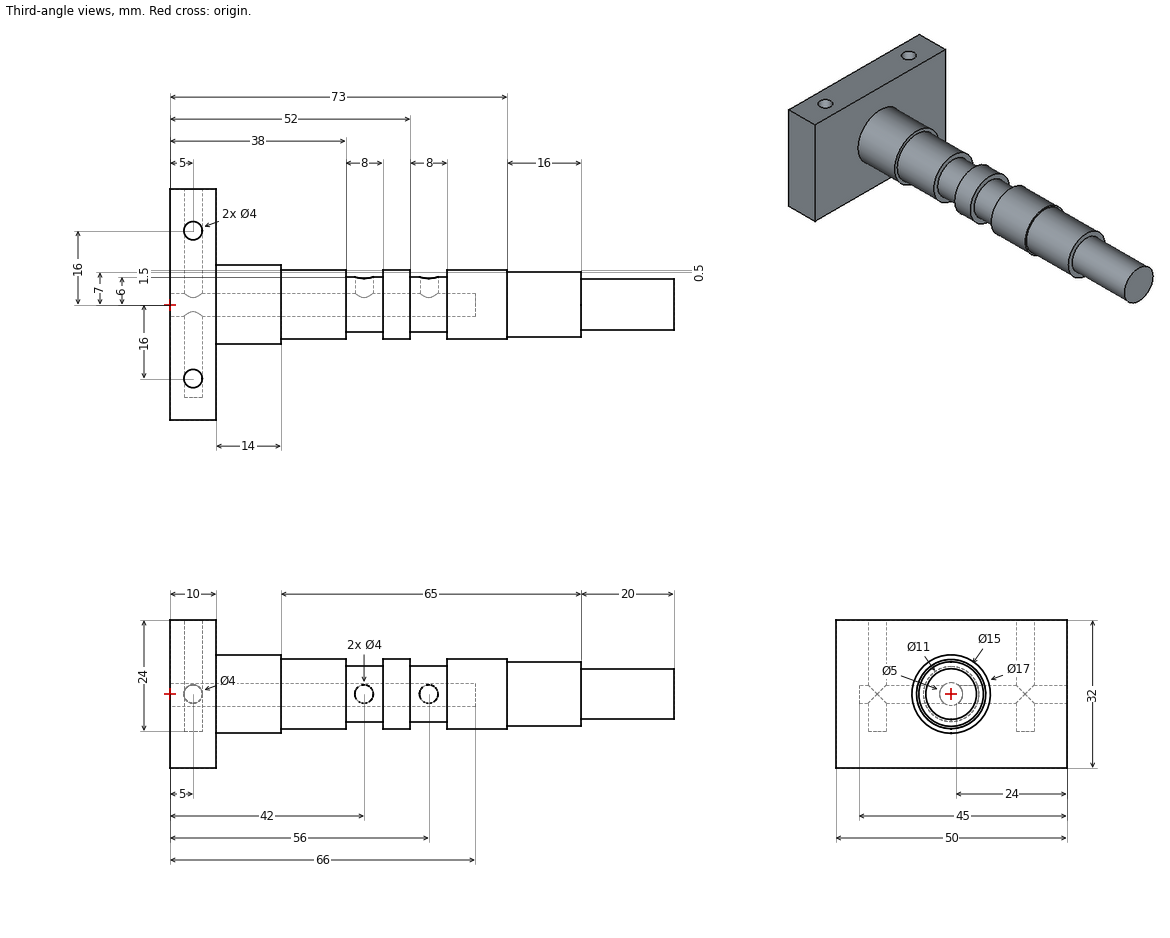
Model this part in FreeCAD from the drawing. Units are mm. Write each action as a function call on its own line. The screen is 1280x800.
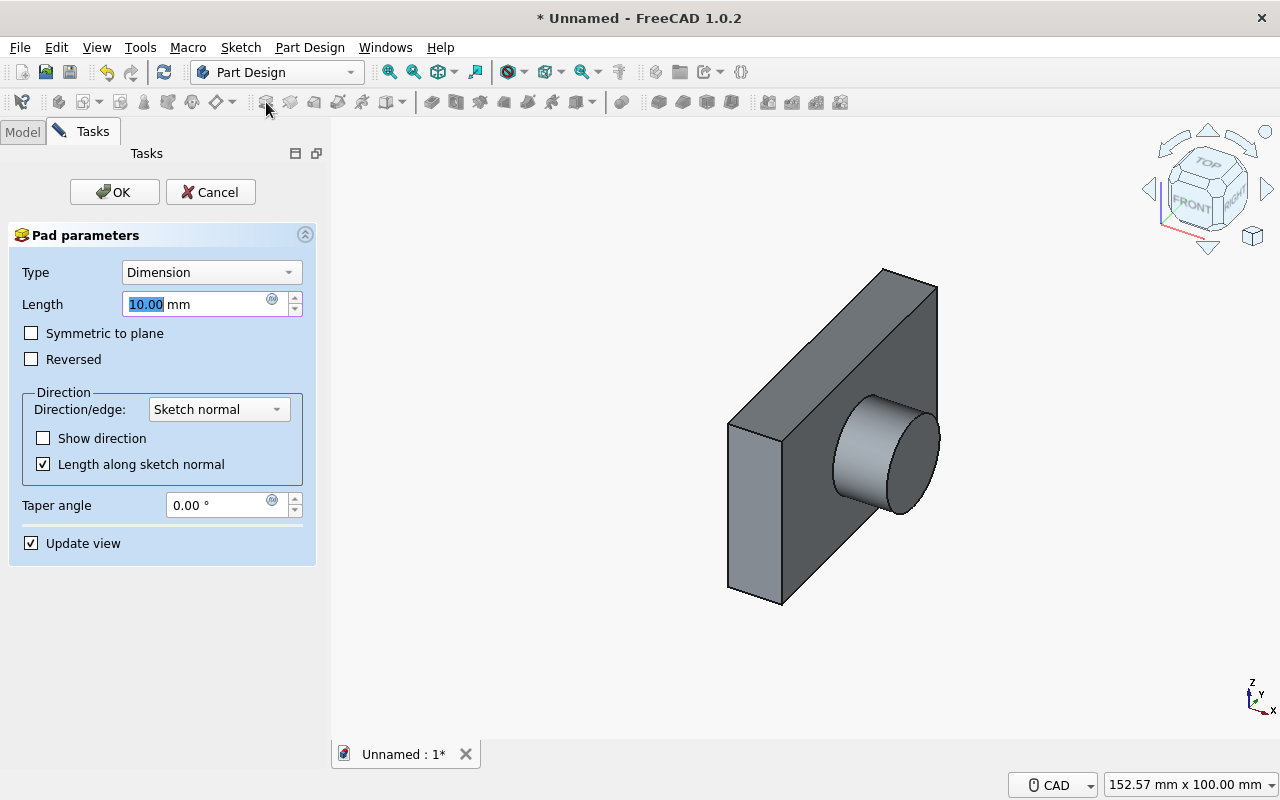
text(14)
key(Tab)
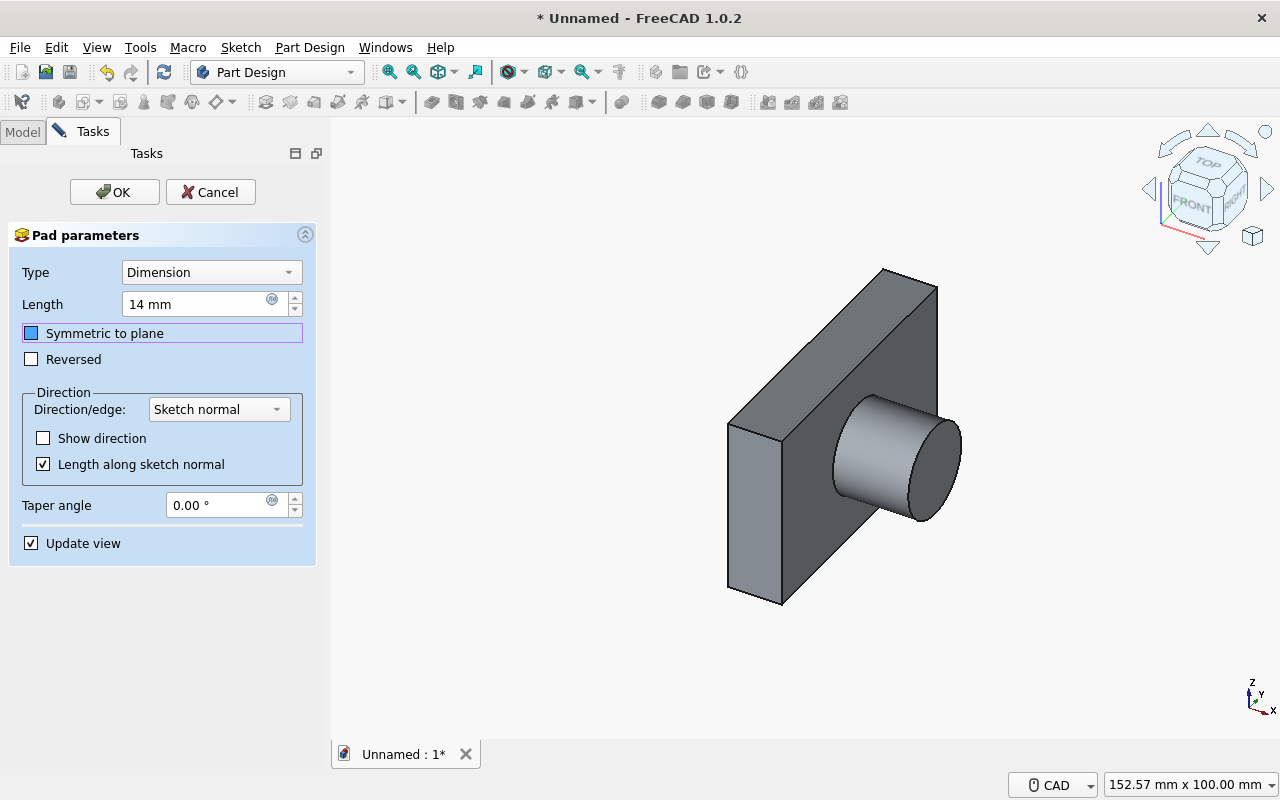
click(115, 192)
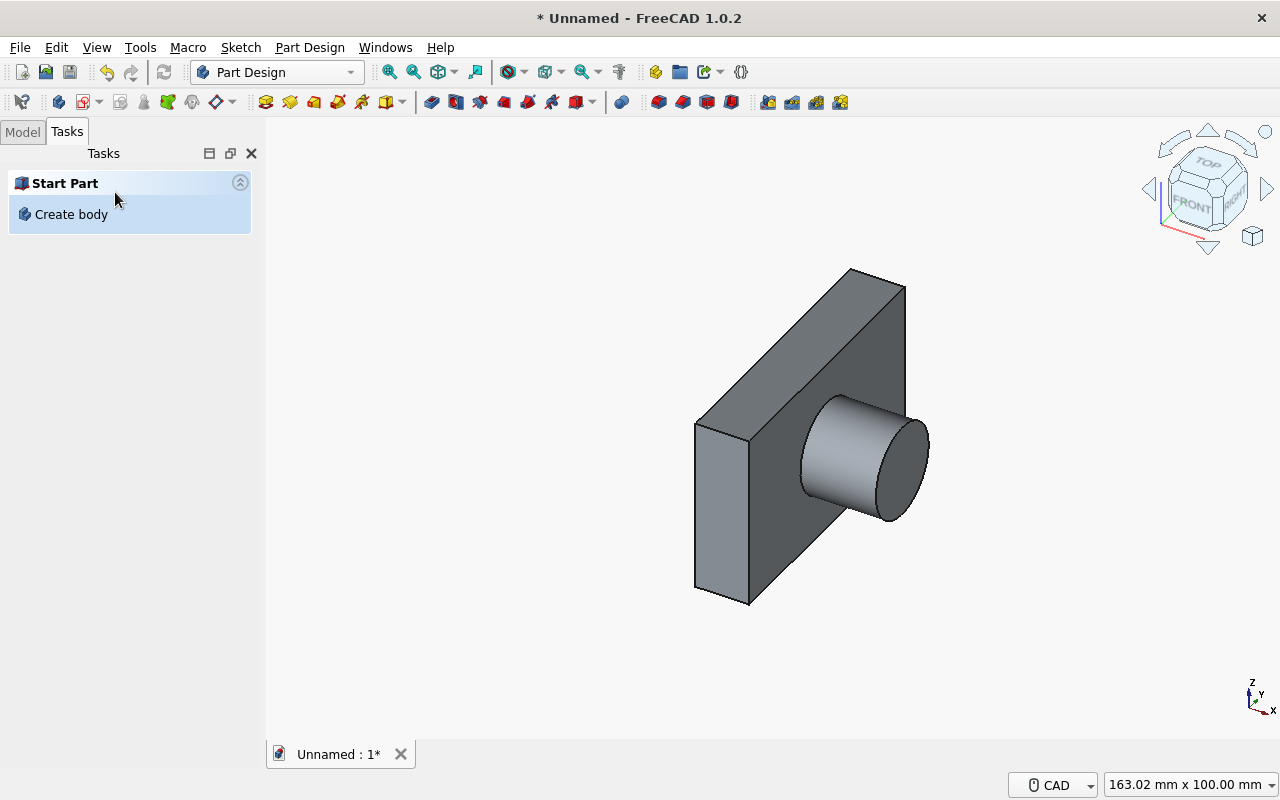
click(844, 310)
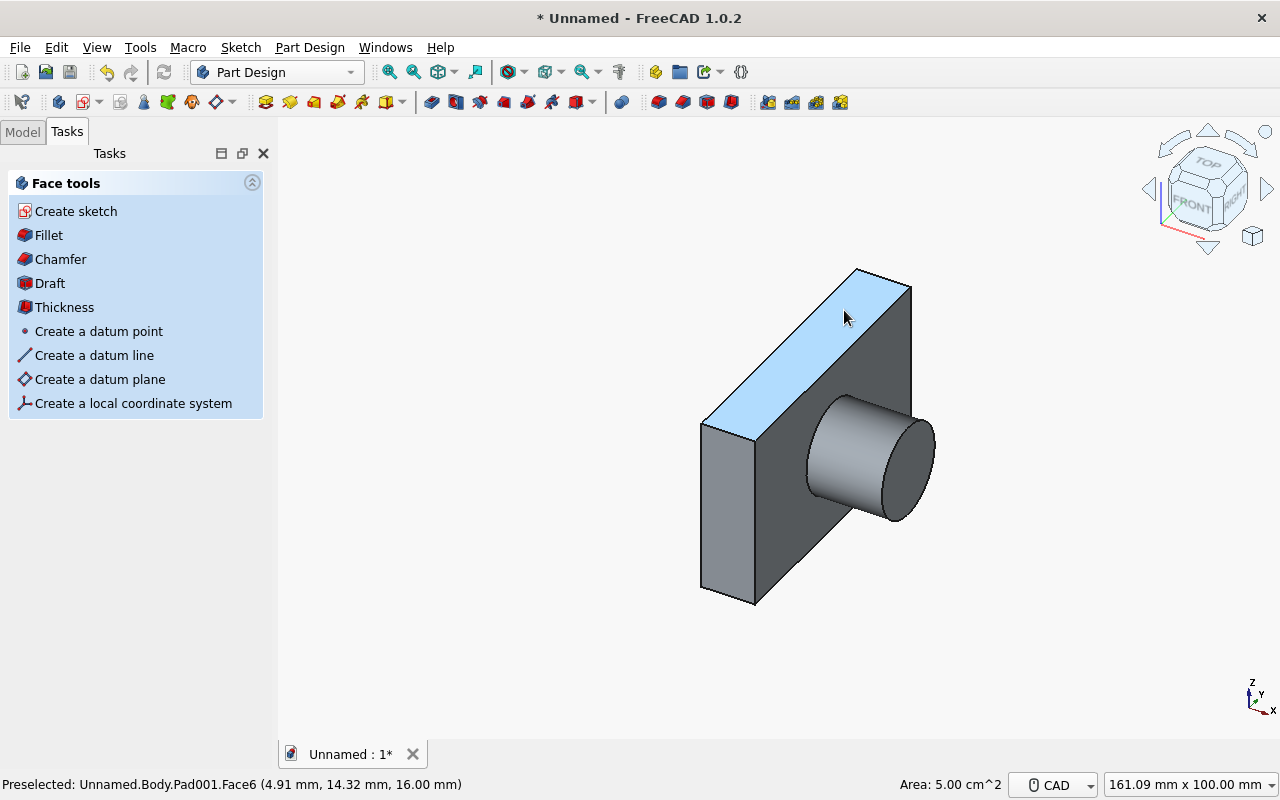
click(84, 102)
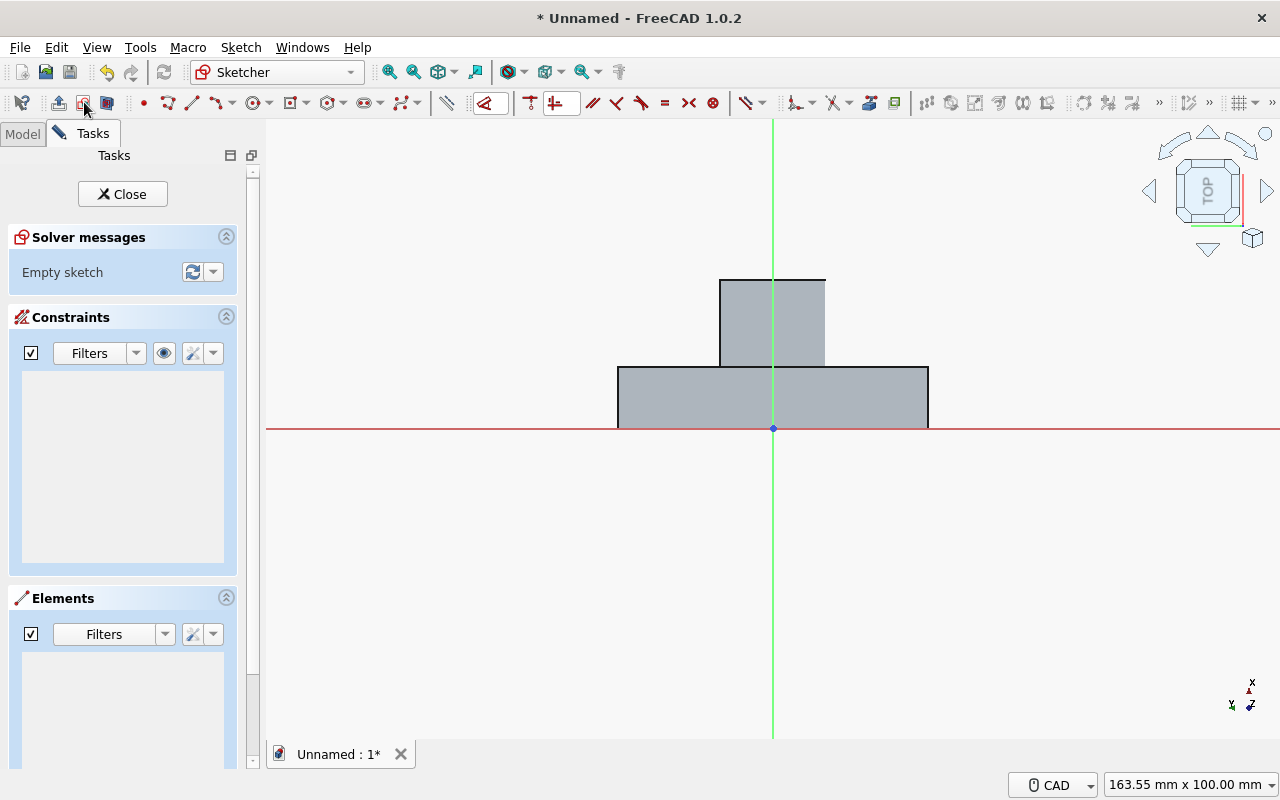
scroll(813, 395, up, 5)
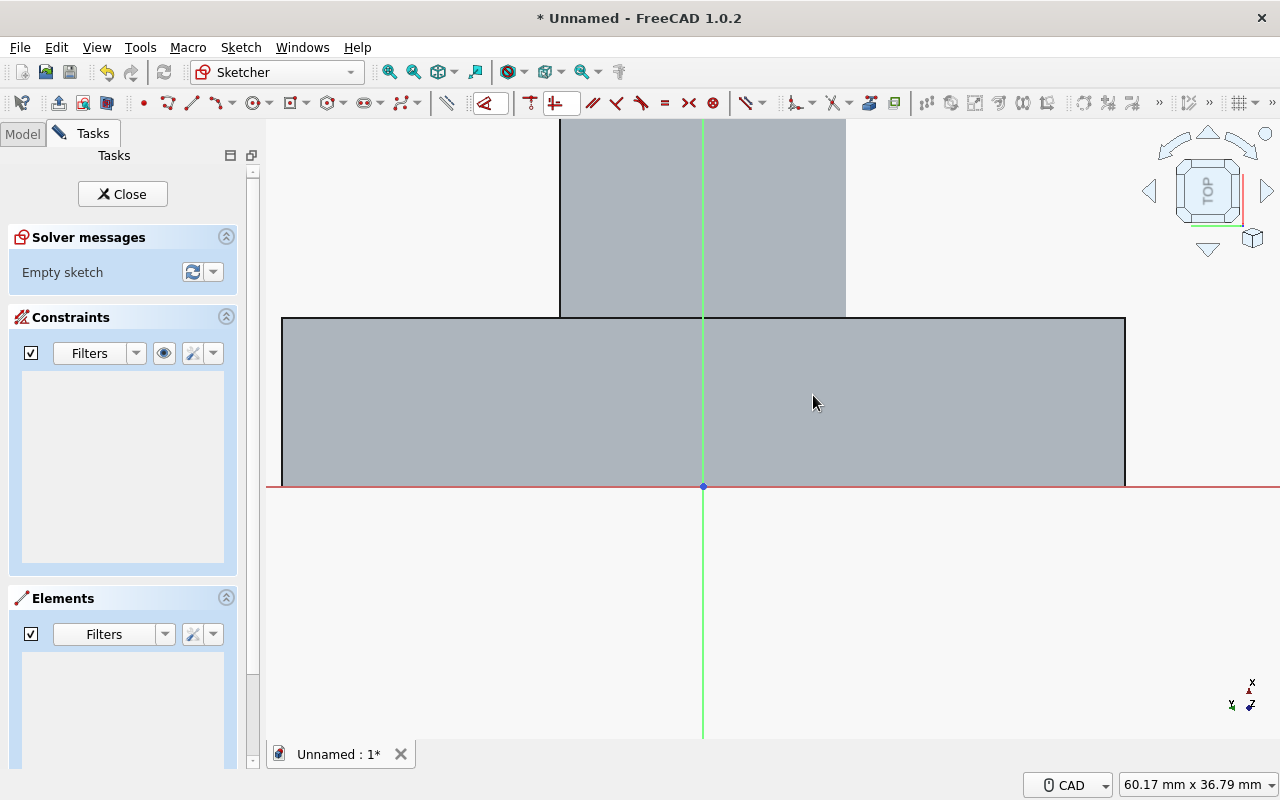
click(254, 104)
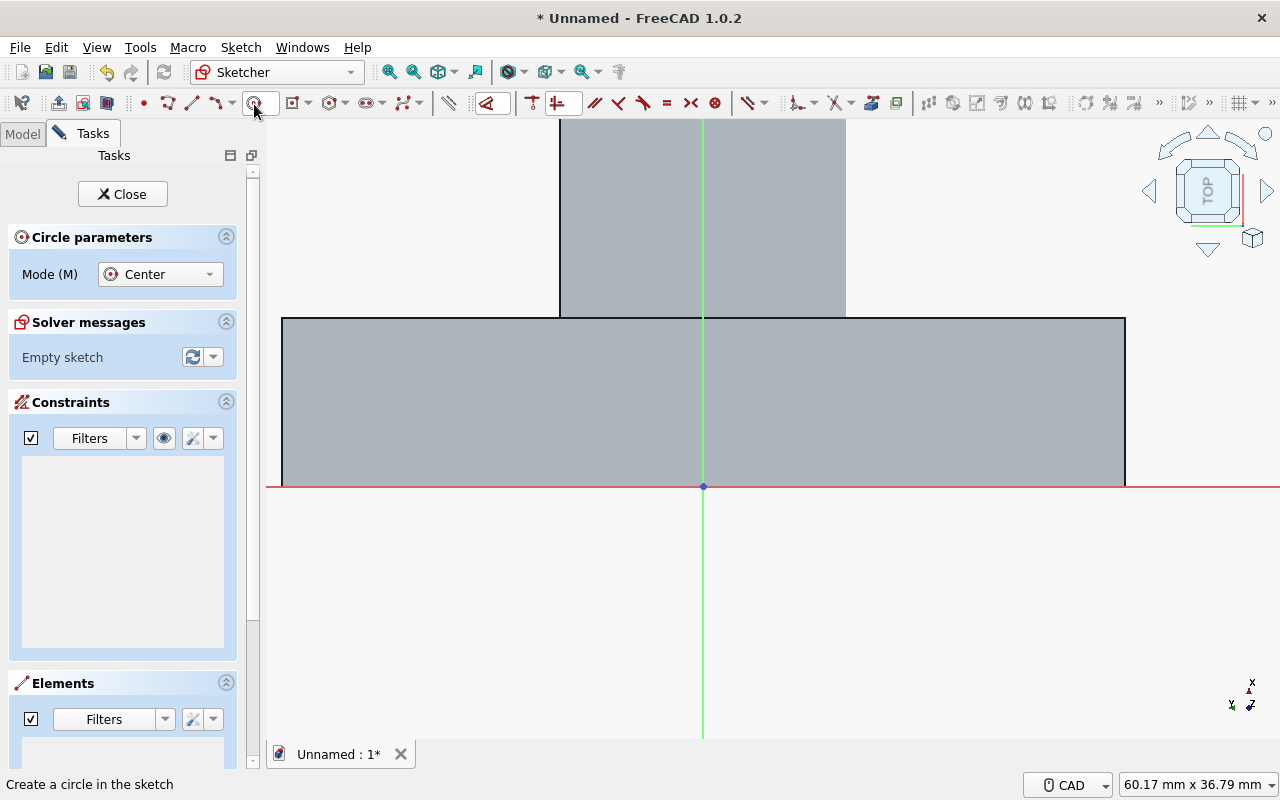
click(434, 402)
move(458, 379)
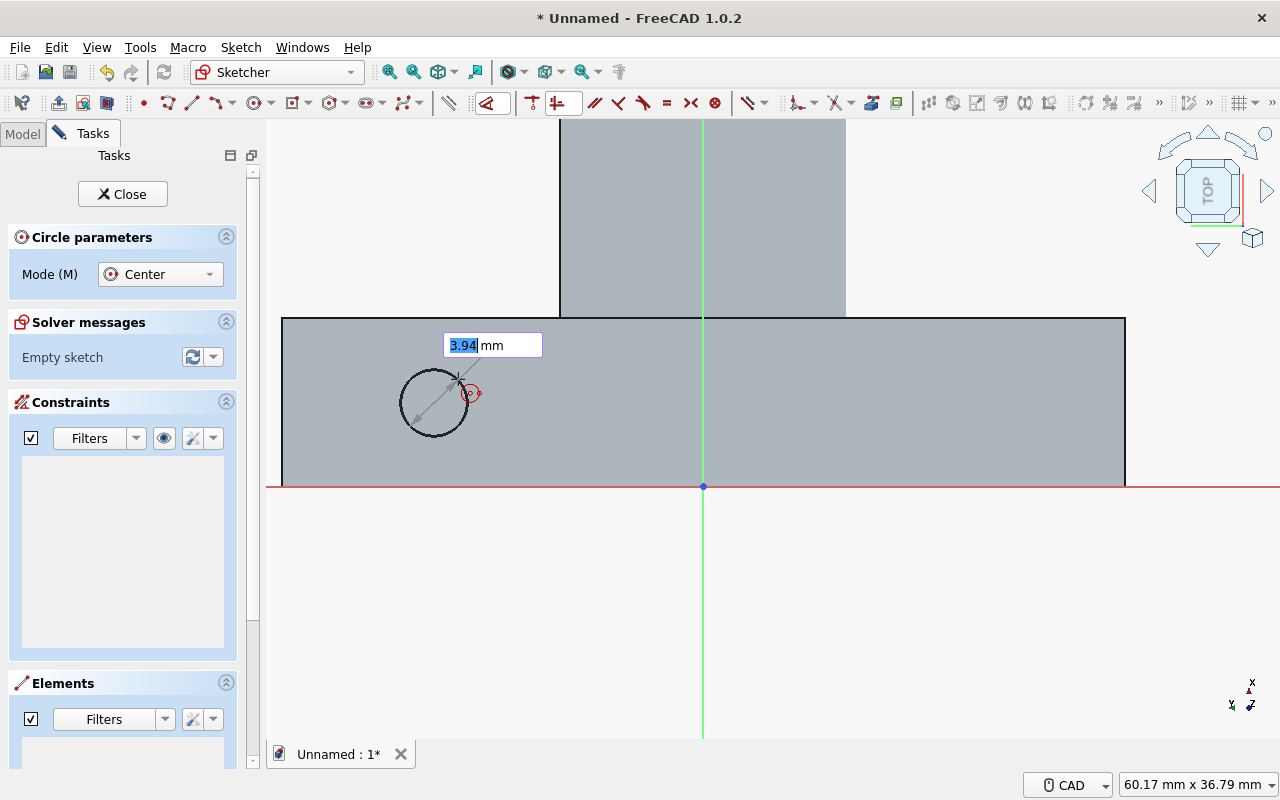
text(4)
key(Return)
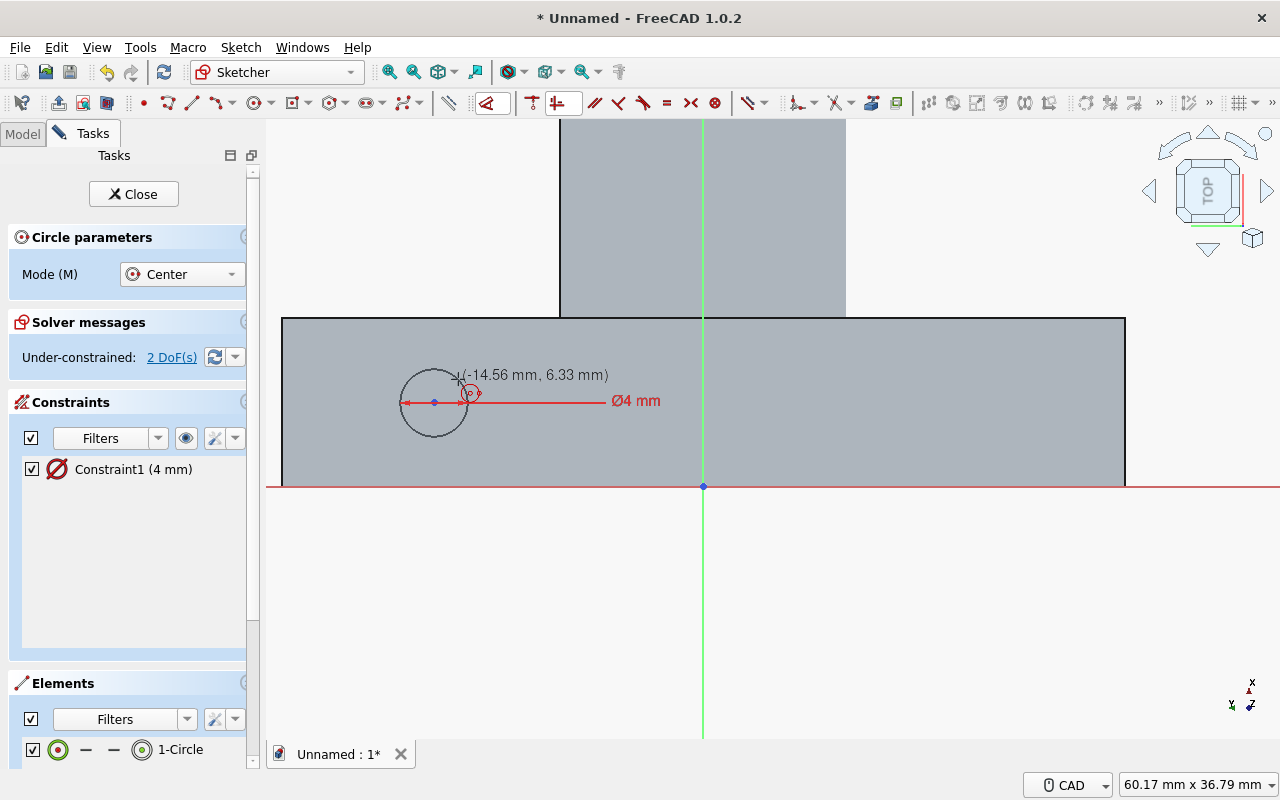
click(973, 402)
move(997, 379)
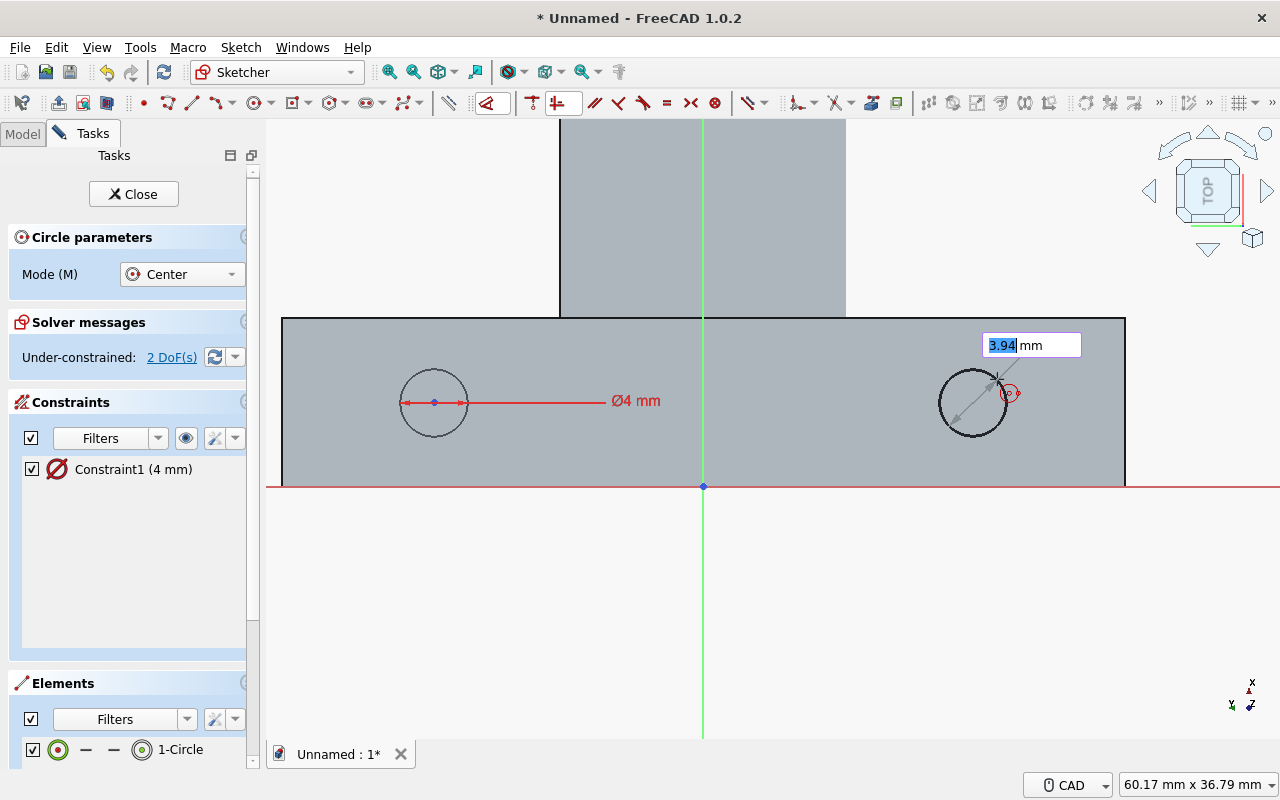
text(4)
key(Return)
key(Escape)